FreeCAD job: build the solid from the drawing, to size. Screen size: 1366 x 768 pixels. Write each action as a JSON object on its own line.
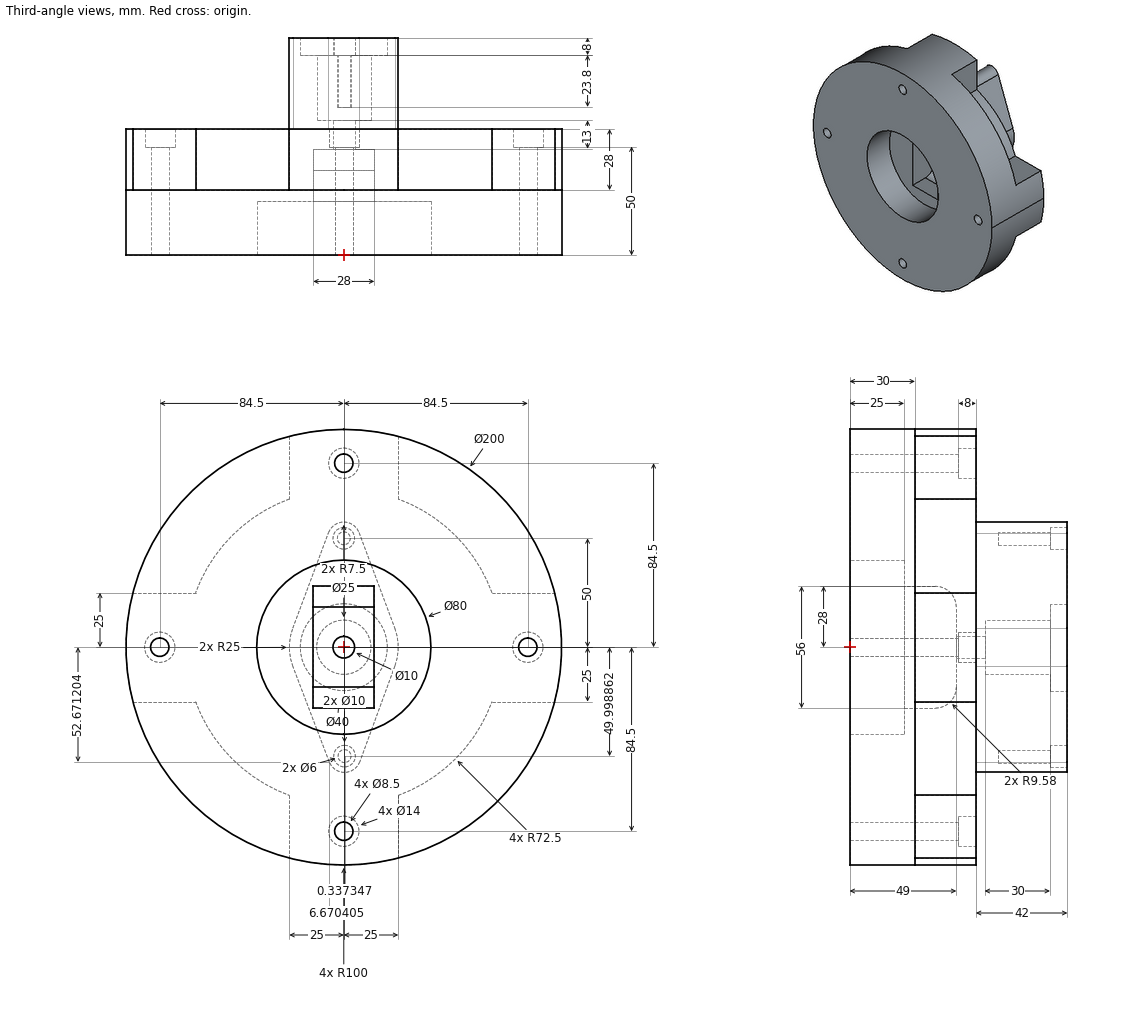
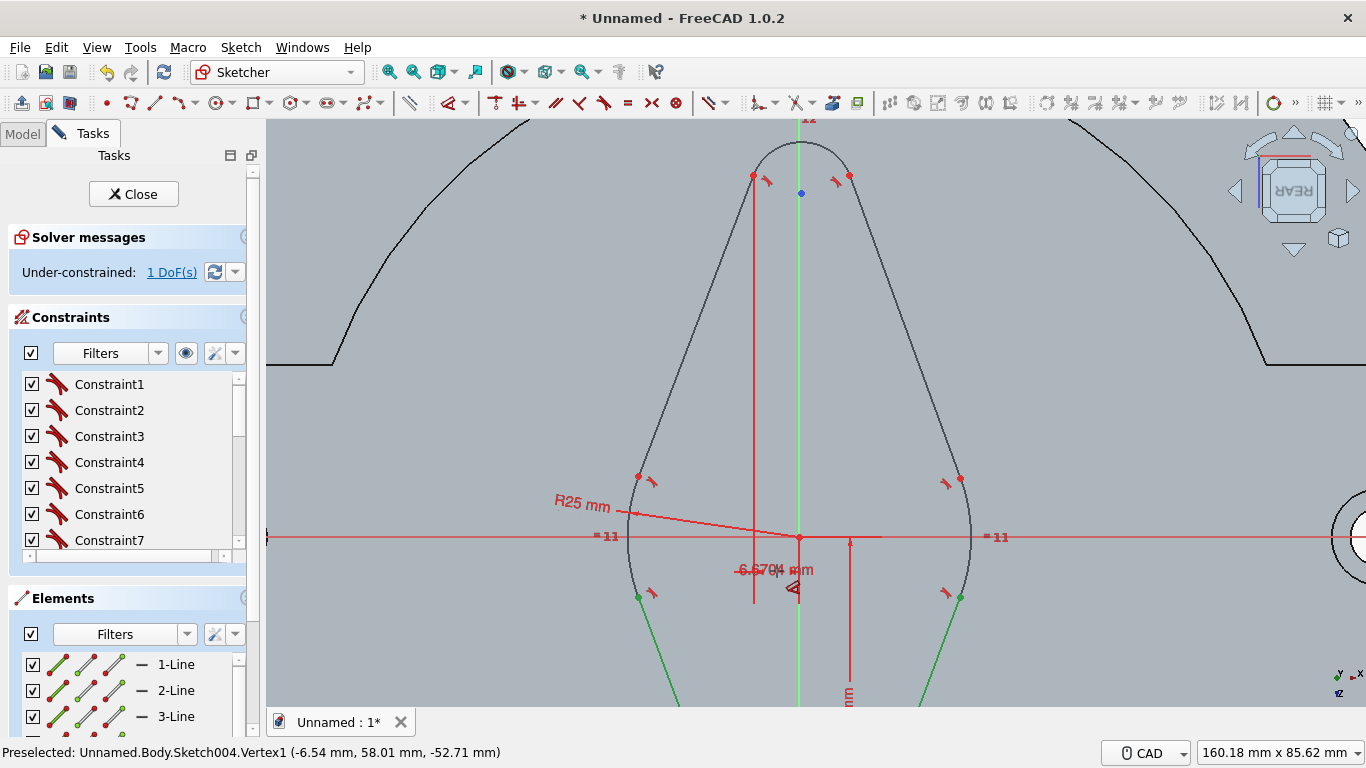
{"action": "left_click", "coordinate": [754, 175]}
{"action": "left_click", "coordinate": [720, 356]}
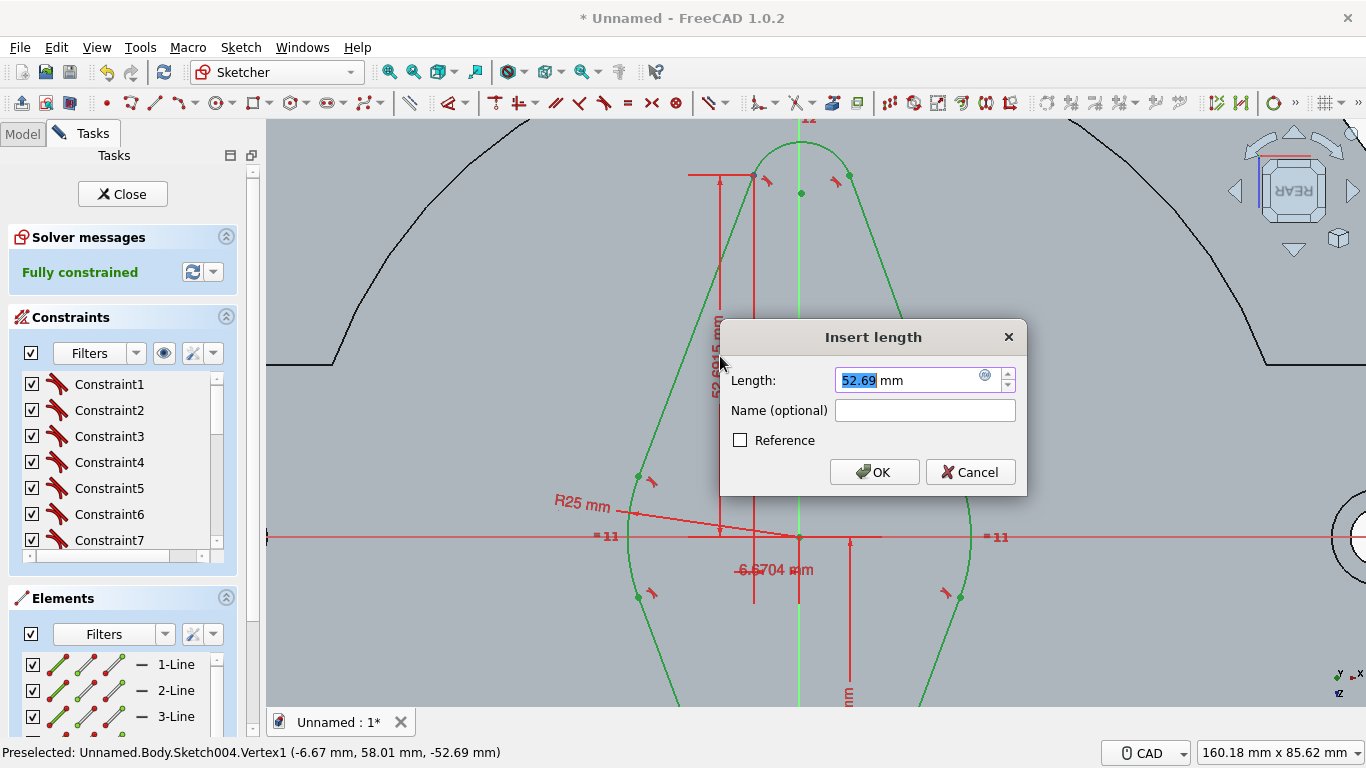
{"action": "type", "text": "52.671204"}
{"action": "key", "text": "Return"}
{"action": "key", "text": "Escape"}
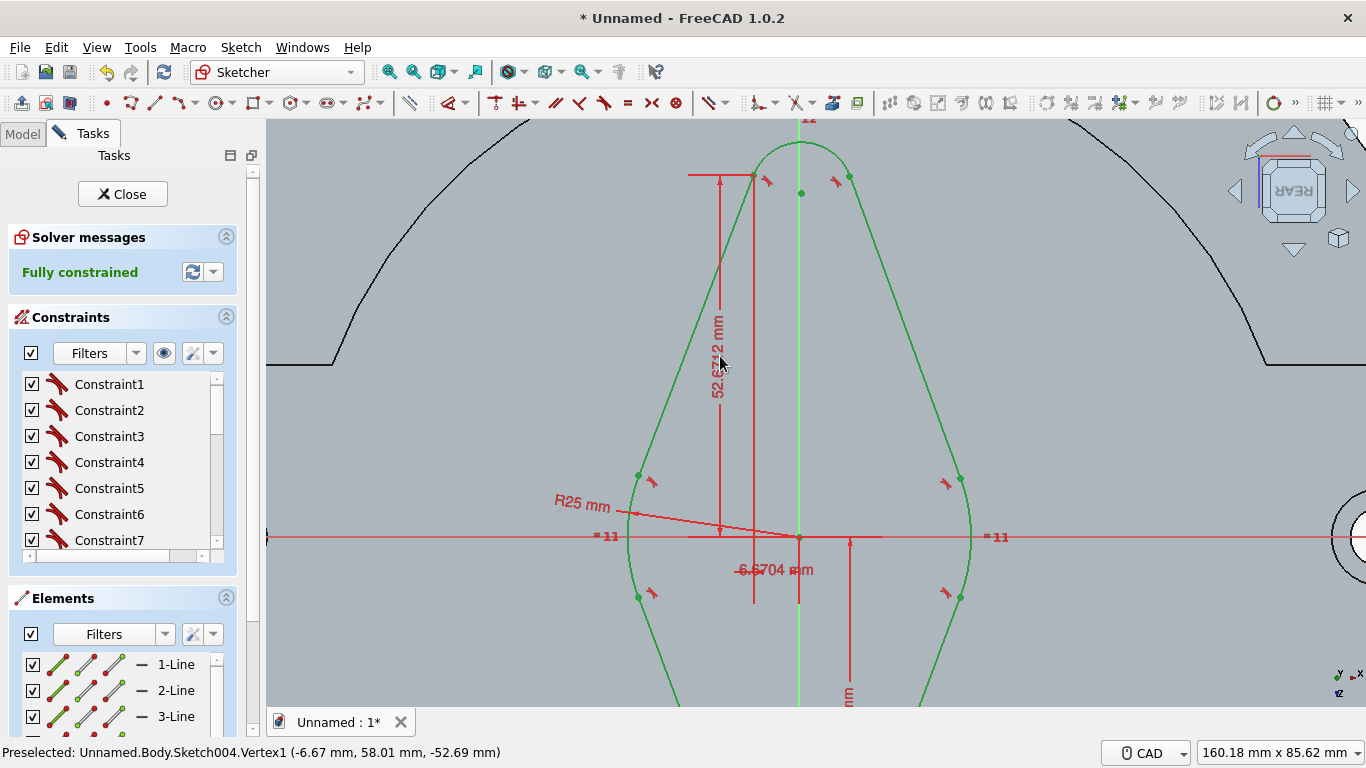
{"action": "left_click", "coordinate": [123, 194]}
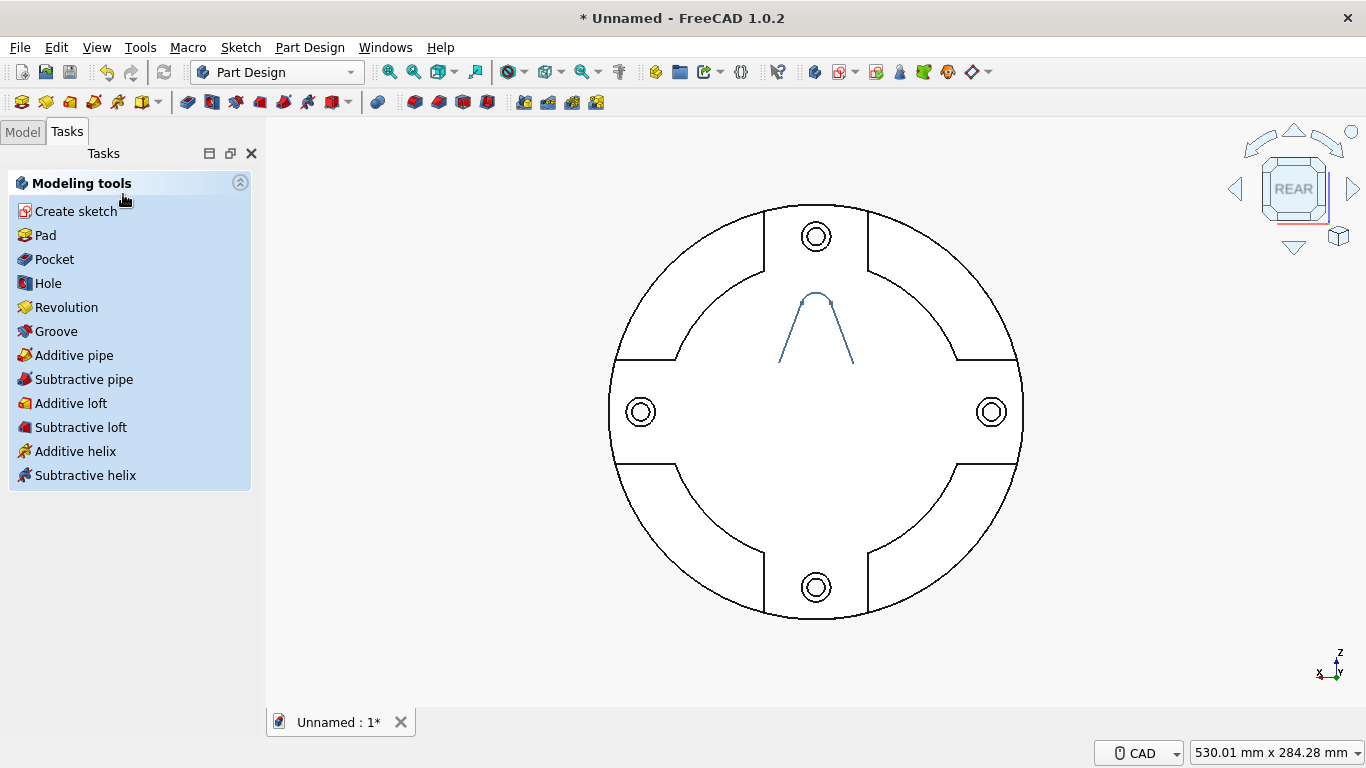
{"action": "left_click", "coordinate": [22, 102]}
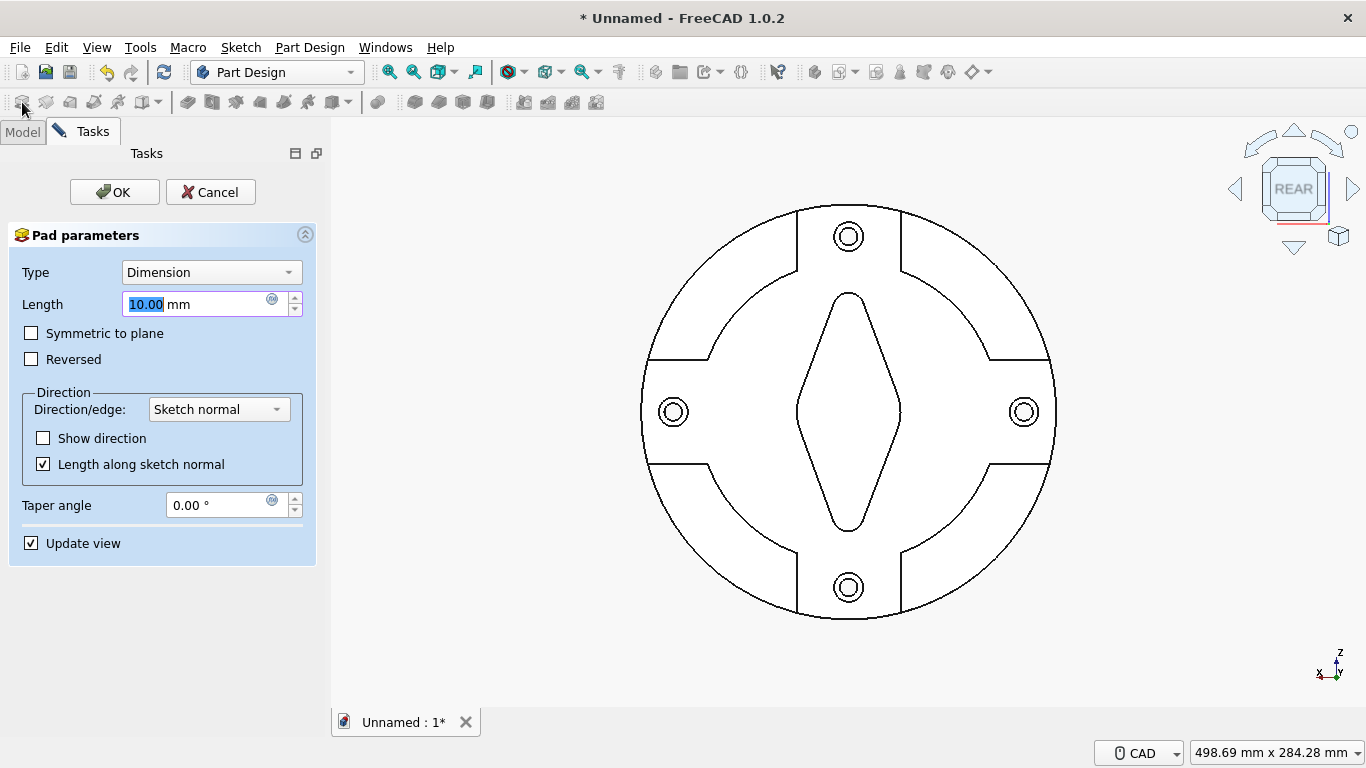
{"action": "type", "text": "42"}
{"action": "key", "text": "Tab"}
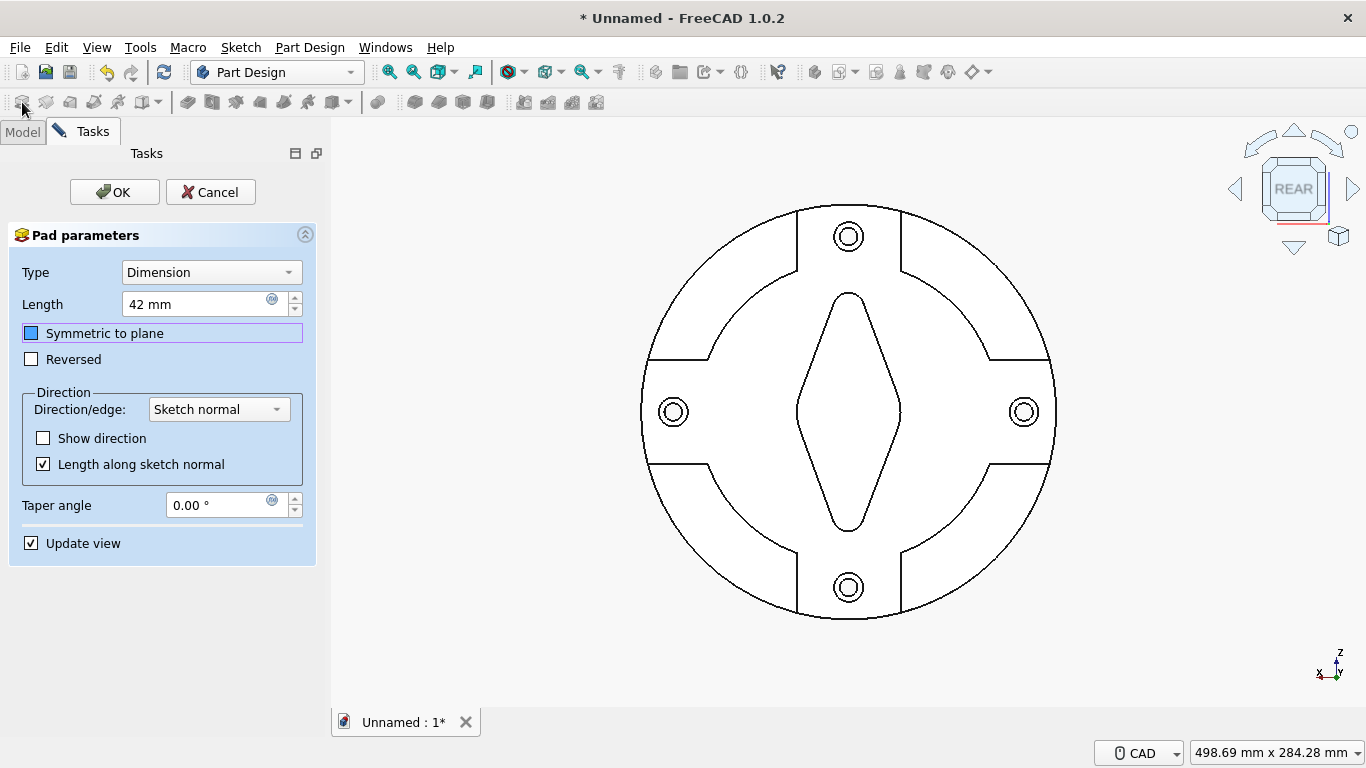
{"action": "left_click", "coordinate": [115, 192]}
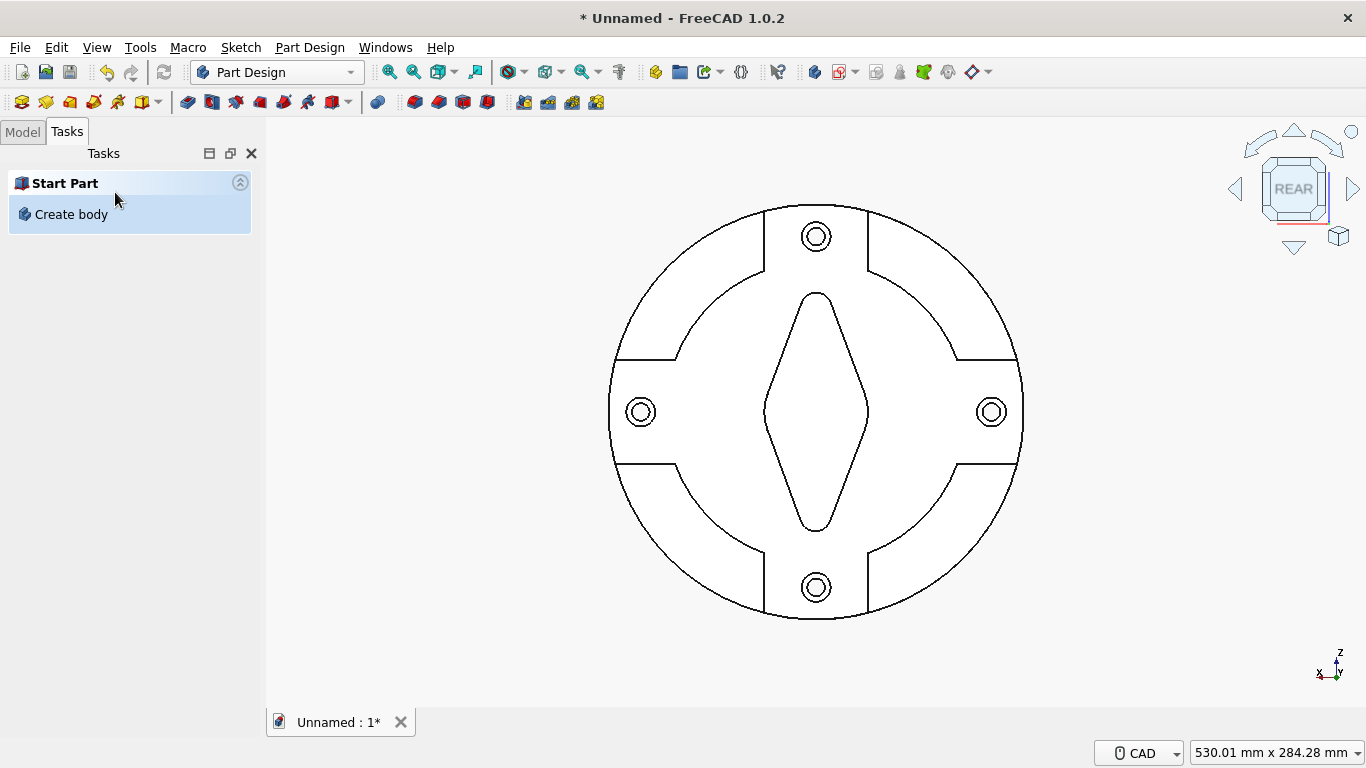
{"action": "left_click", "coordinate": [816, 411]}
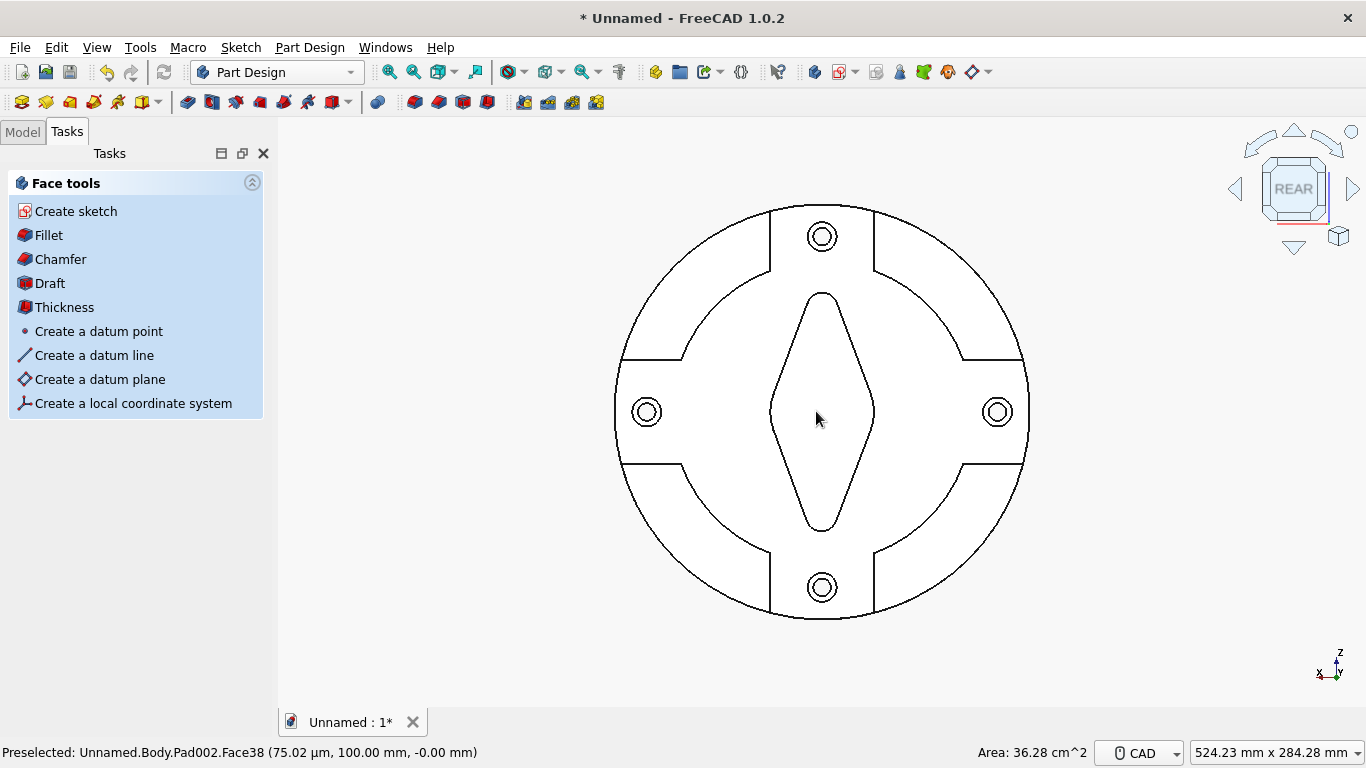
{"action": "left_click", "coordinate": [840, 72]}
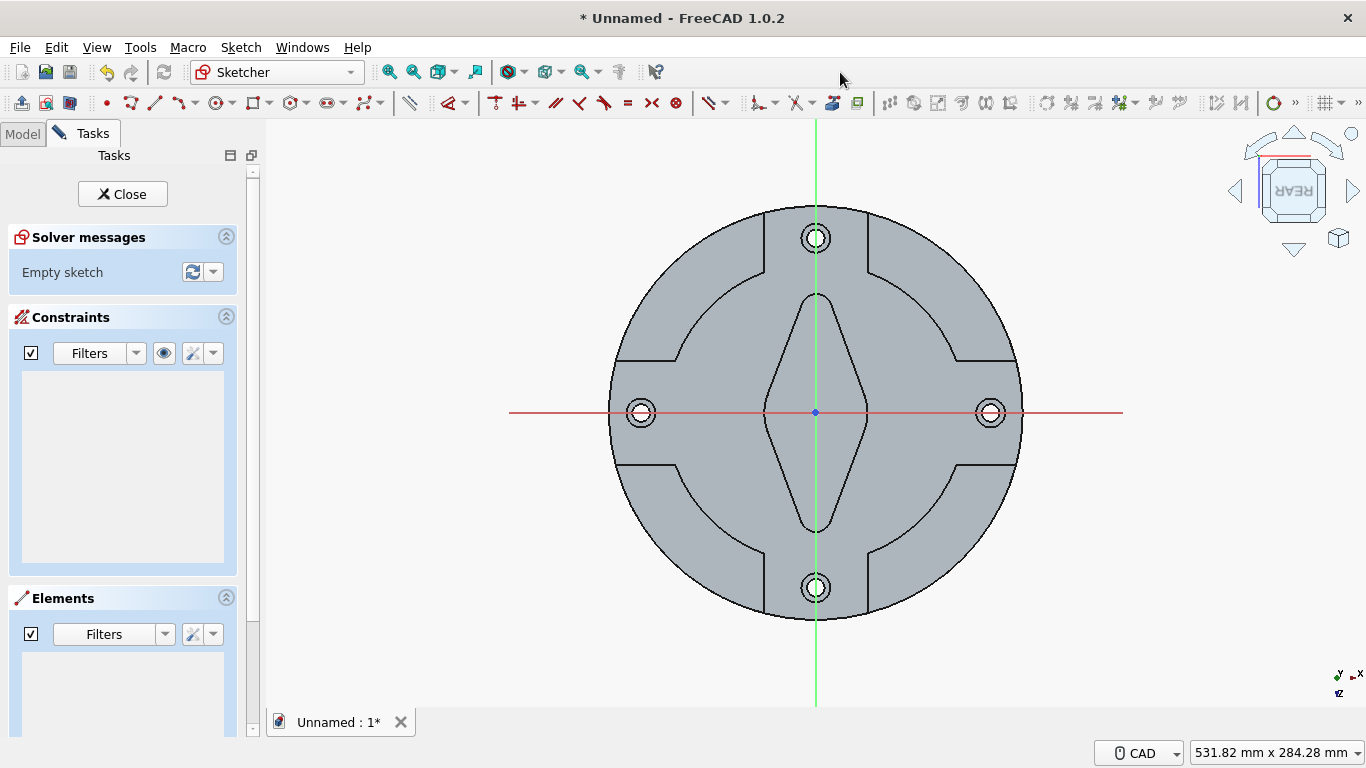
{"action": "scroll", "coordinate": [833, 413], "scroll_direction": "up", "scroll_amount": 8}